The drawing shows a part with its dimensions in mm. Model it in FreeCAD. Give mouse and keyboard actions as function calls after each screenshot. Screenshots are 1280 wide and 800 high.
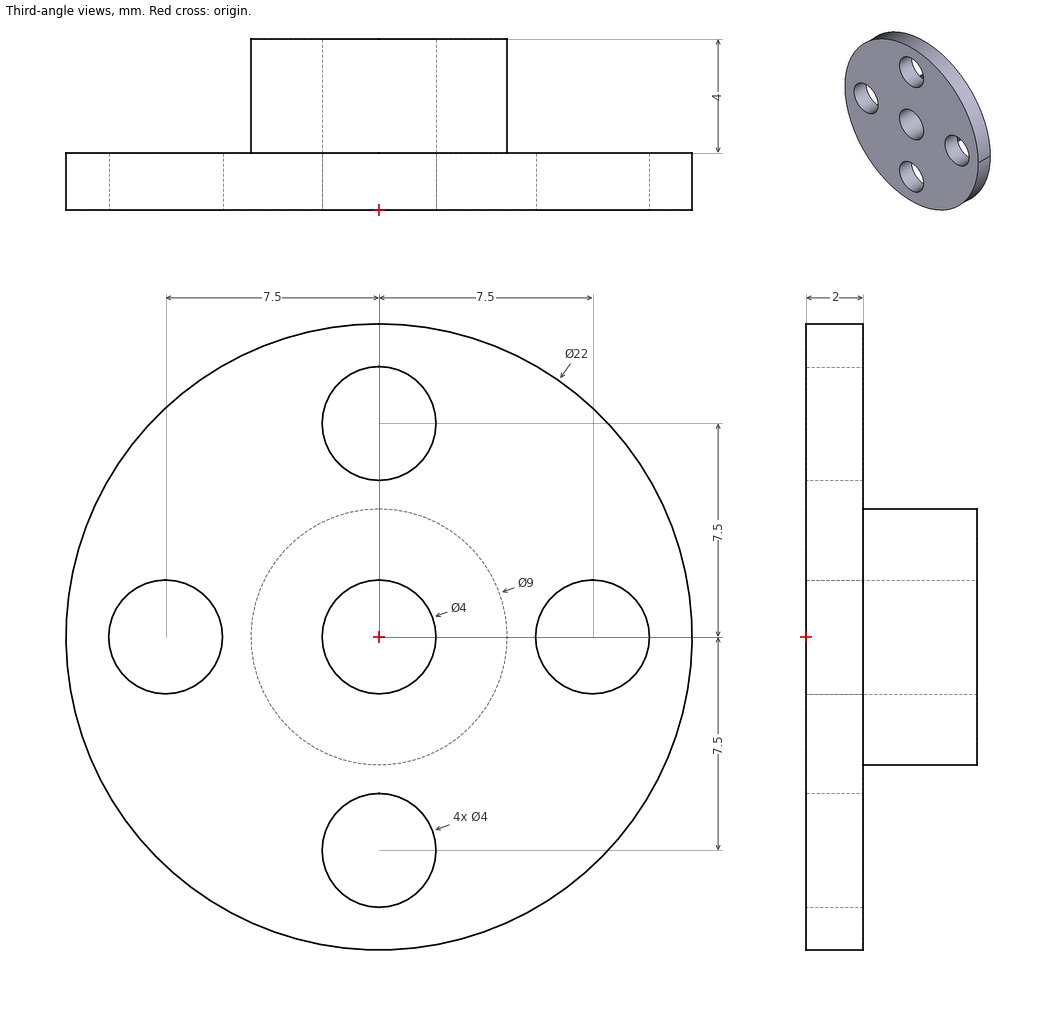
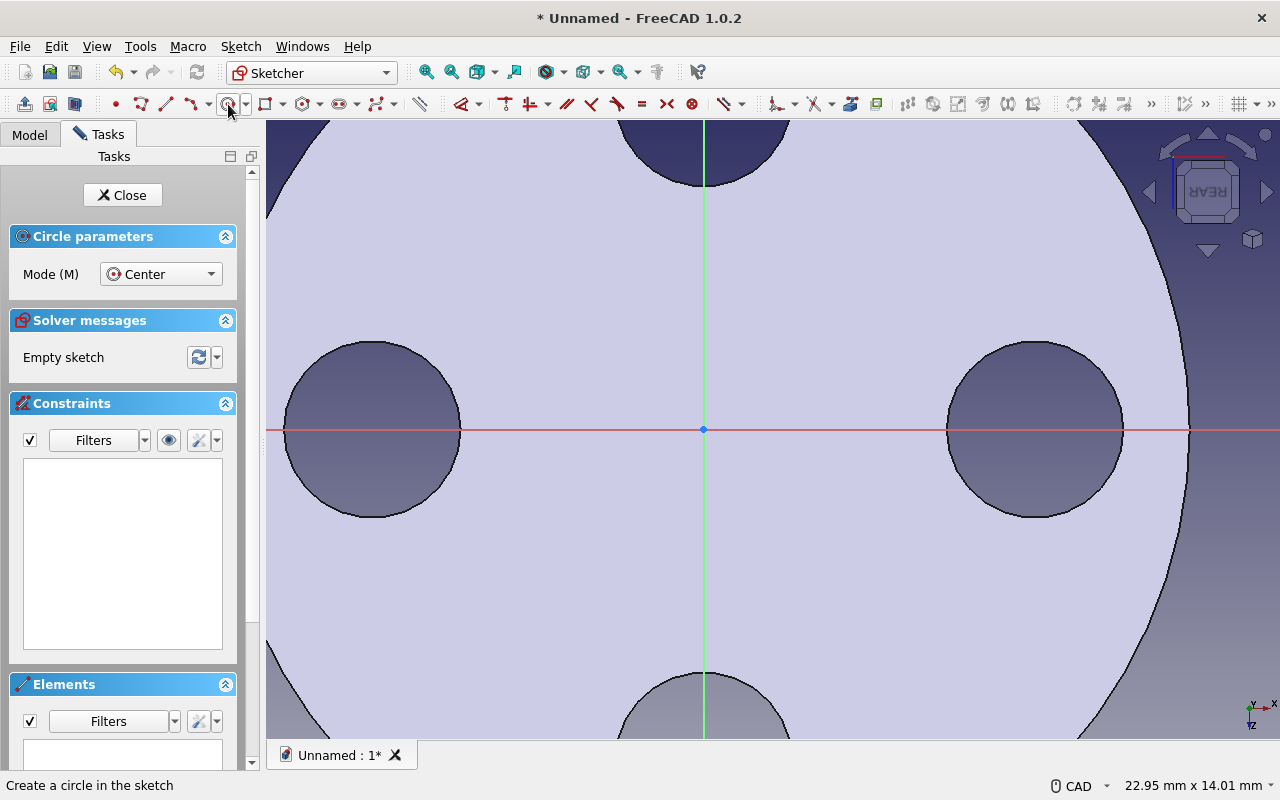
click(704, 429)
click(844, 289)
key(Escape)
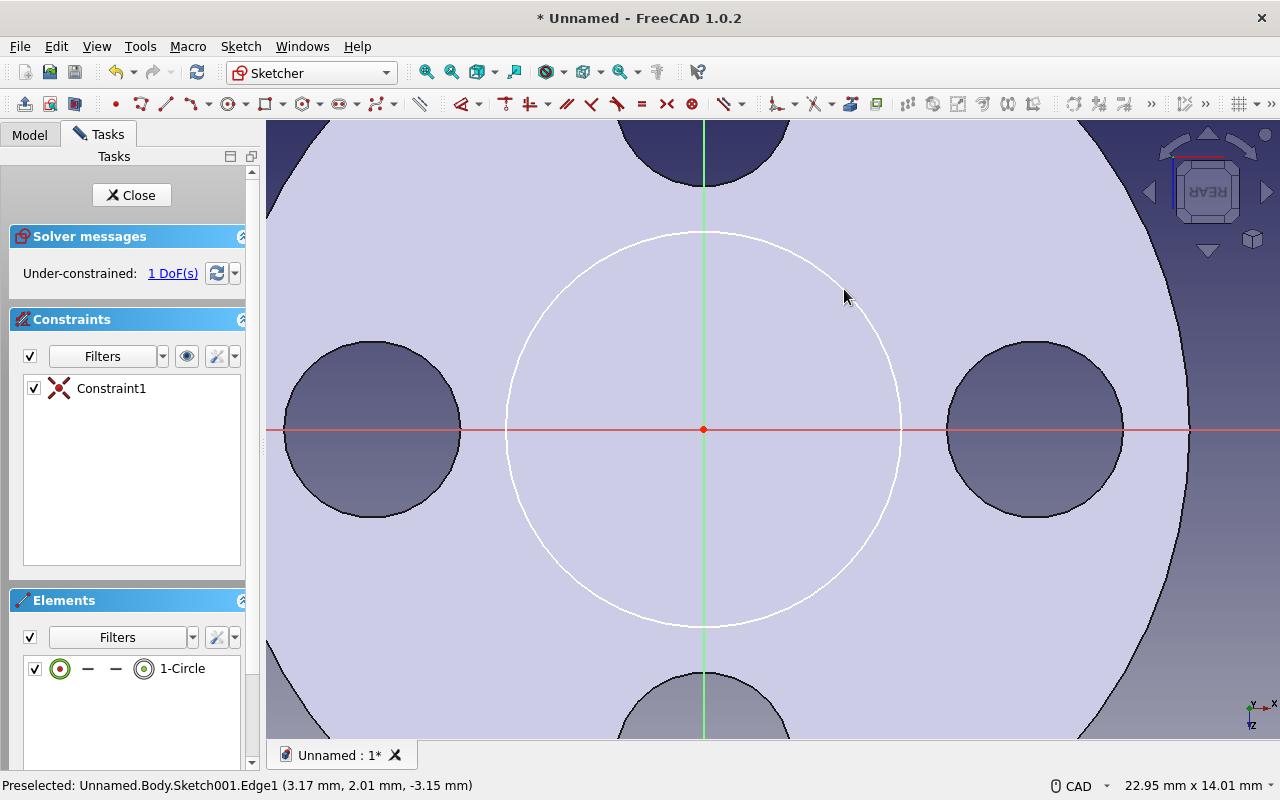
click(460, 104)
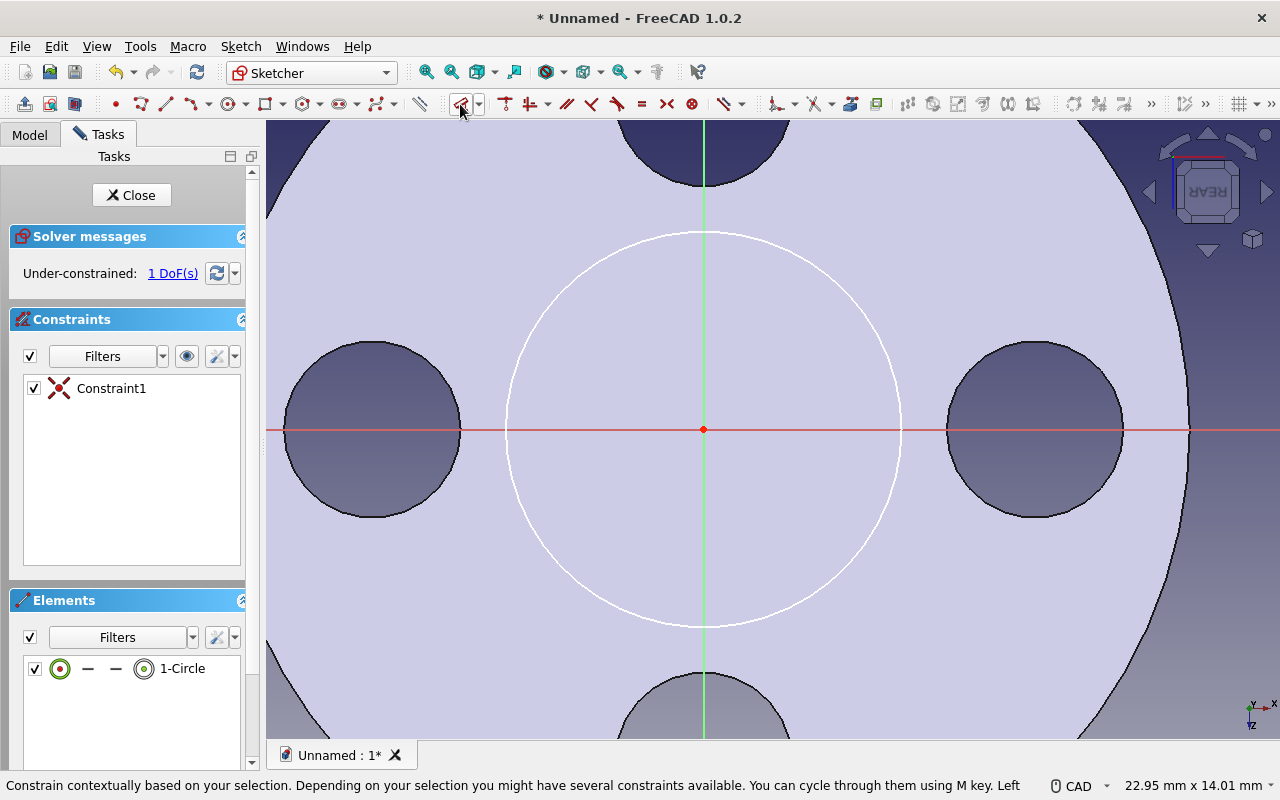
click(843, 289)
click(866, 266)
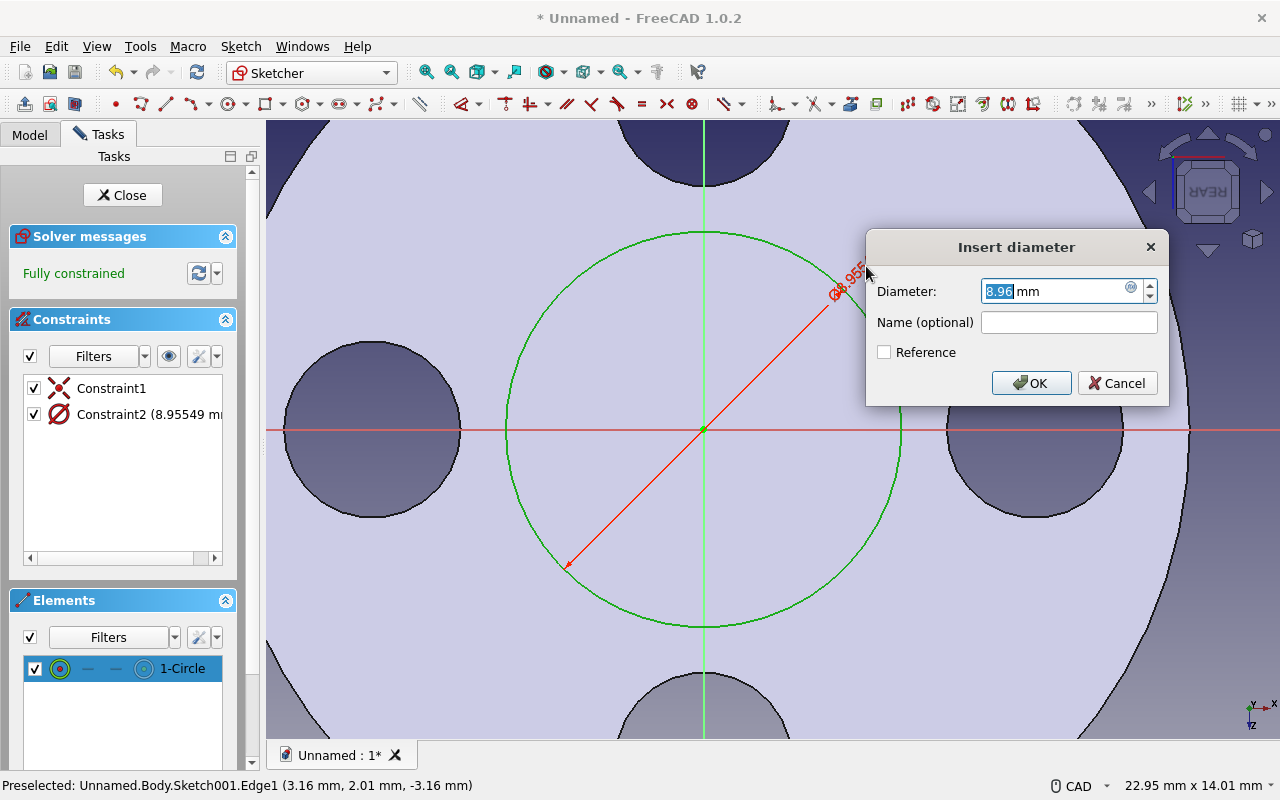
text(9)
key(Return)
key(Escape)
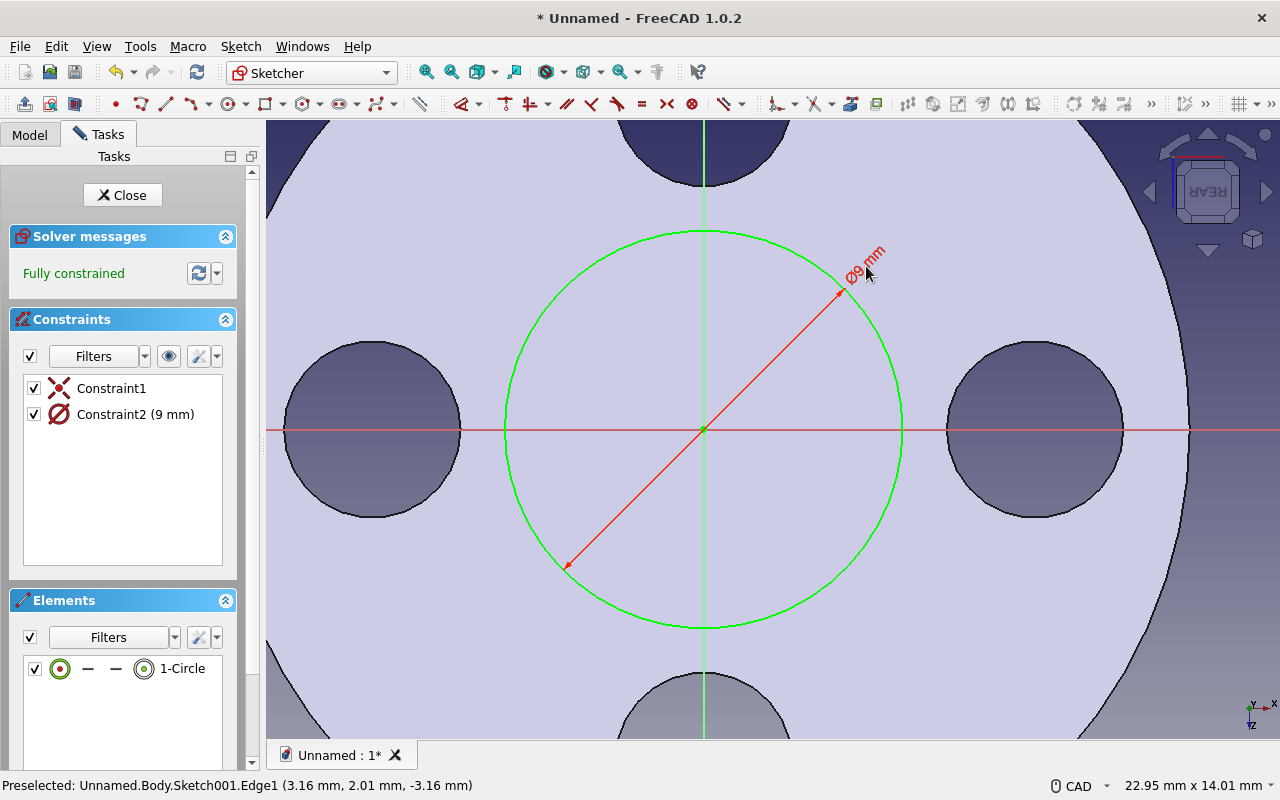
click(123, 195)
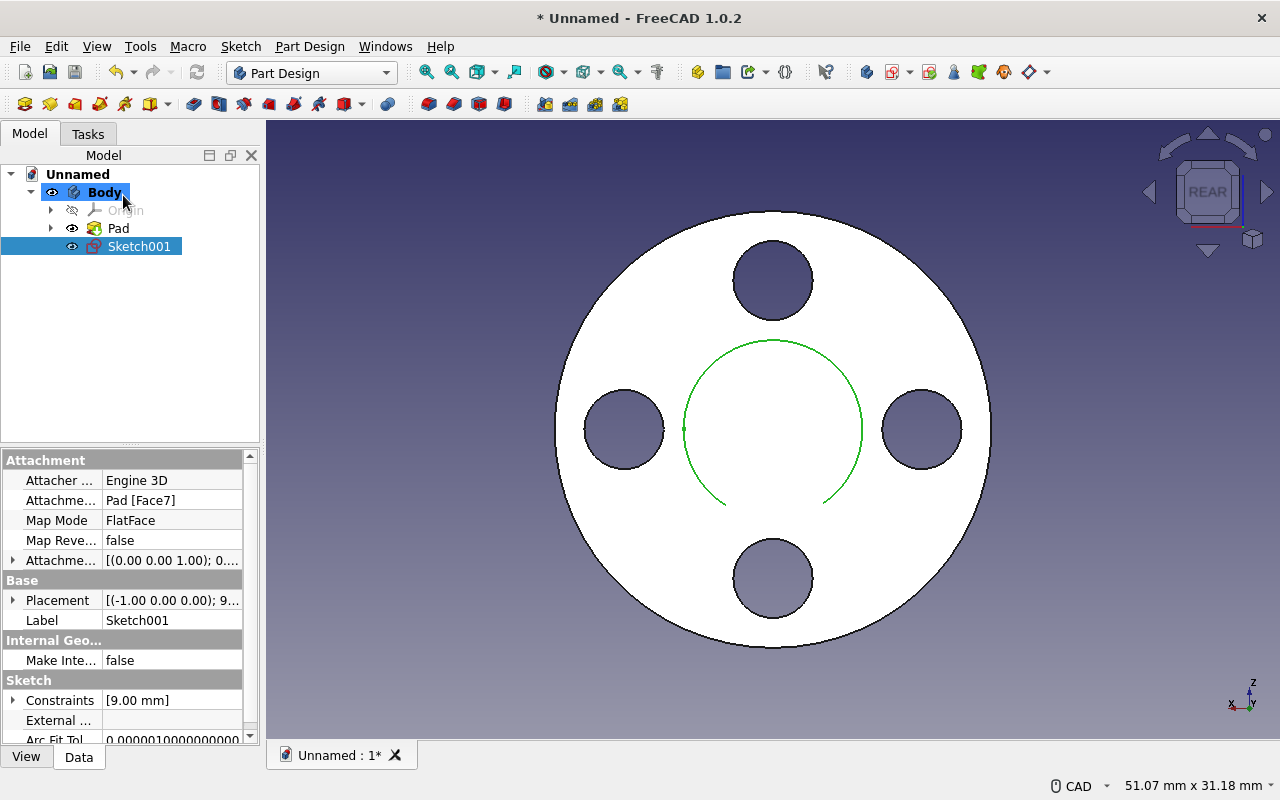
click(25, 104)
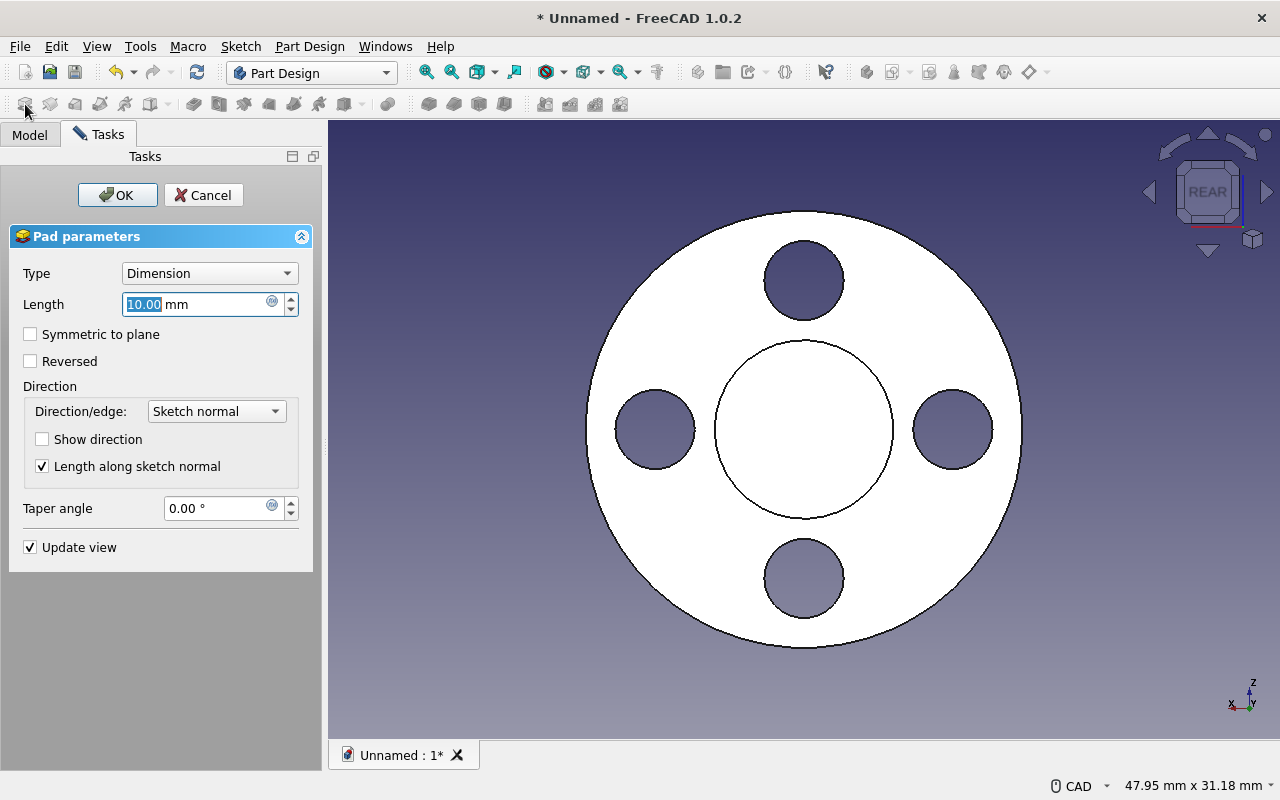
text(4)
key(Tab)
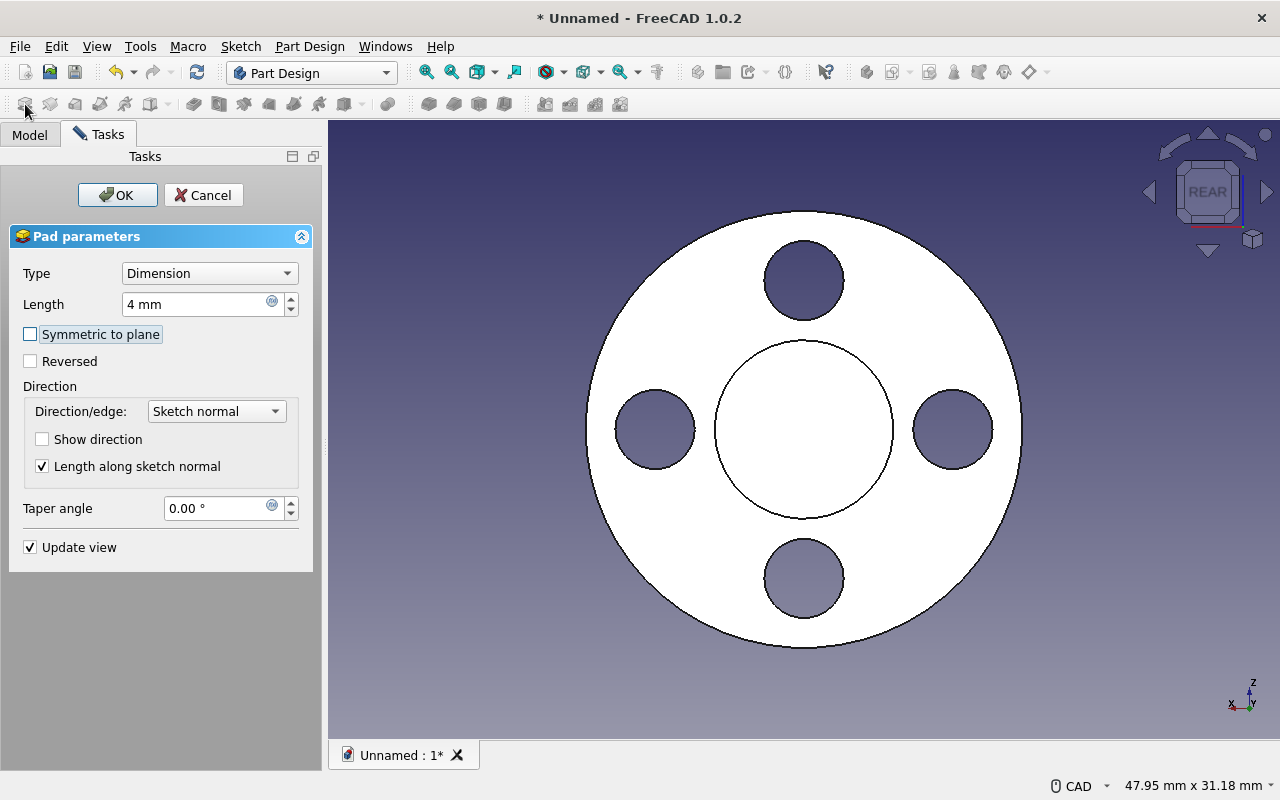
click(118, 195)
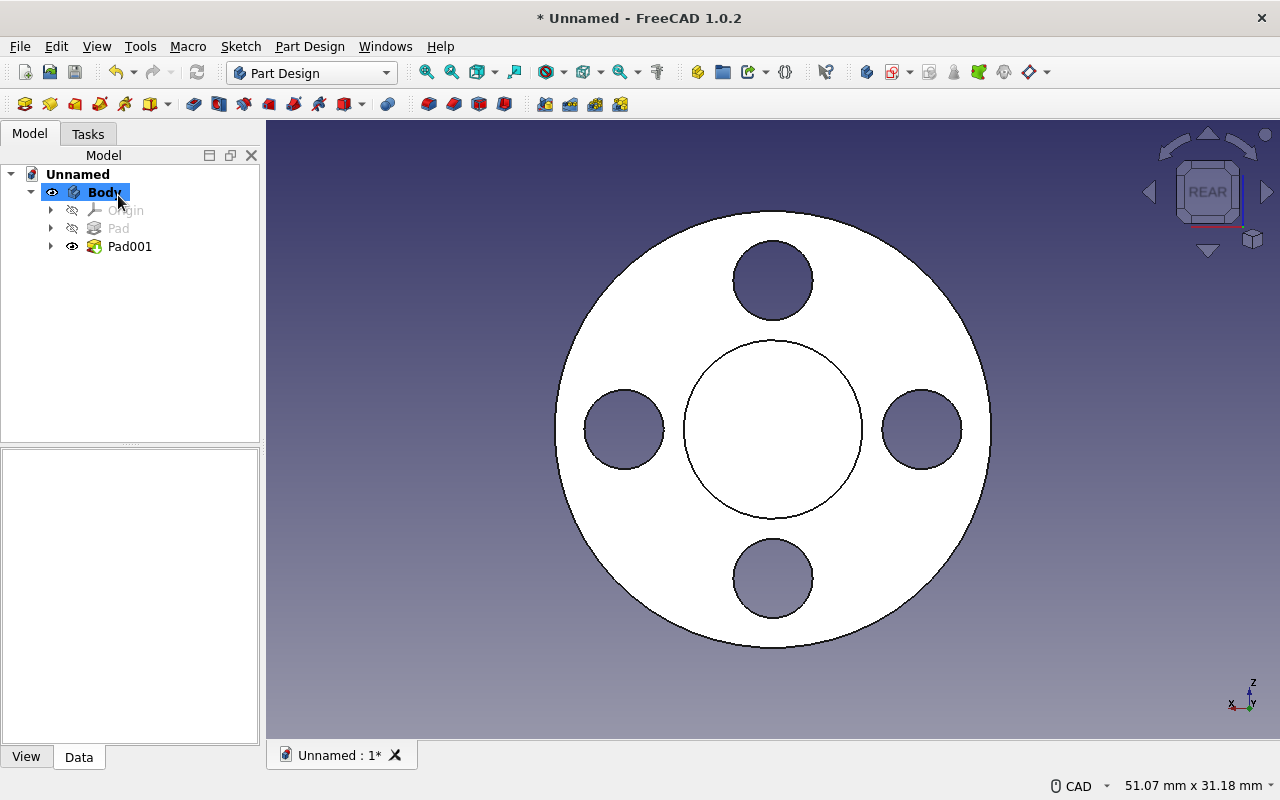
click(773, 429)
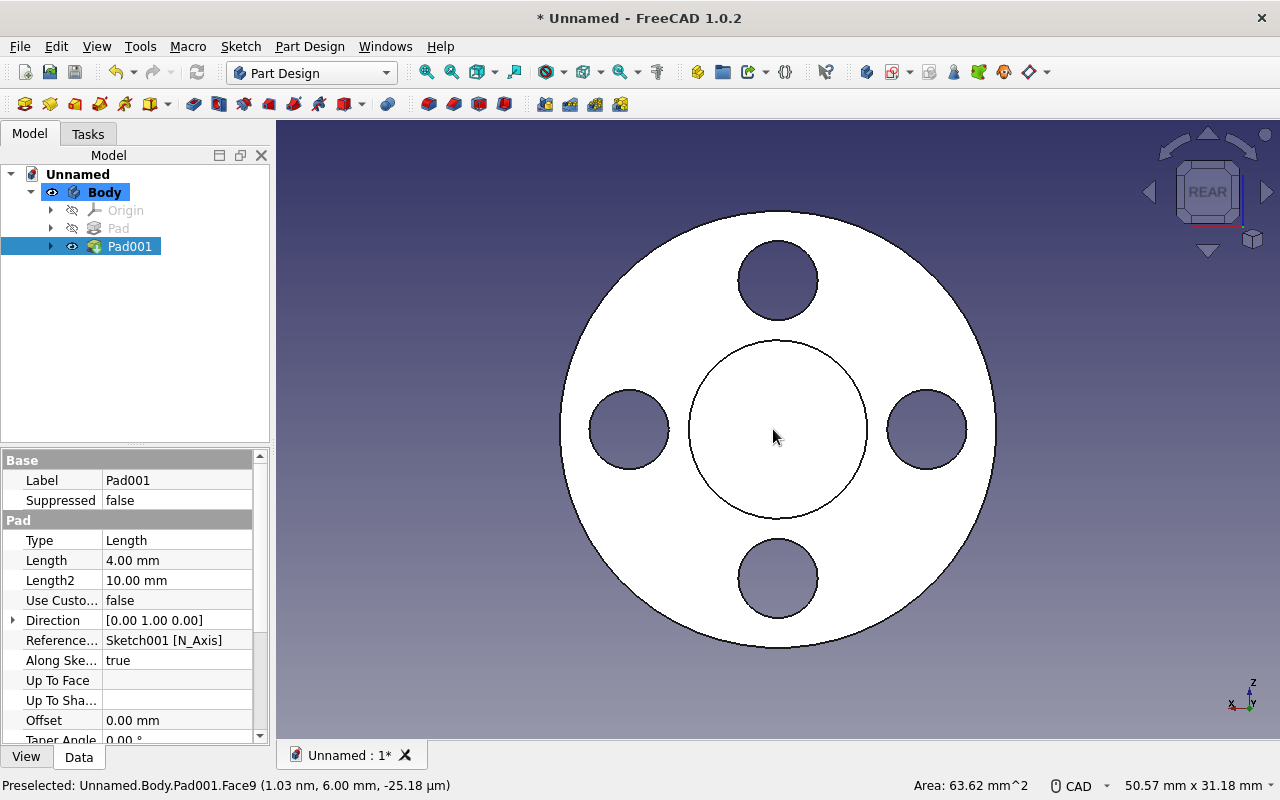
click(892, 72)